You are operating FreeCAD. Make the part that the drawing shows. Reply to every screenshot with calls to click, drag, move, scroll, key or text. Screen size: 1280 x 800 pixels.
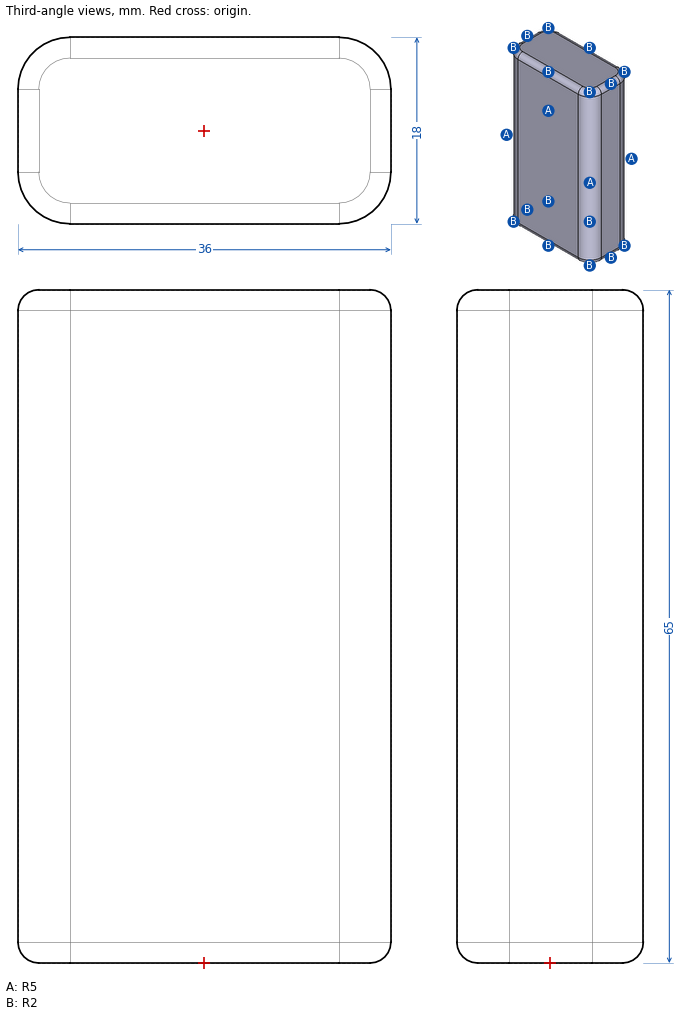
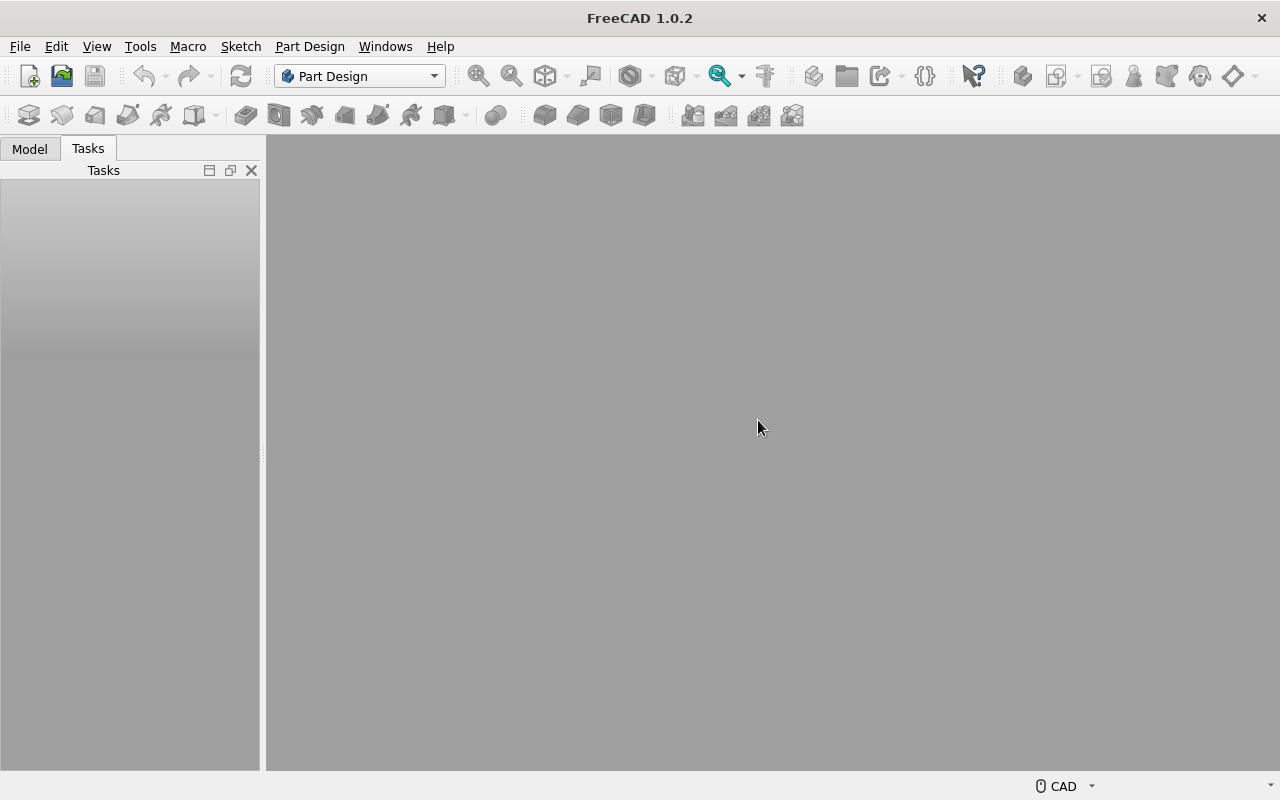
click(29, 76)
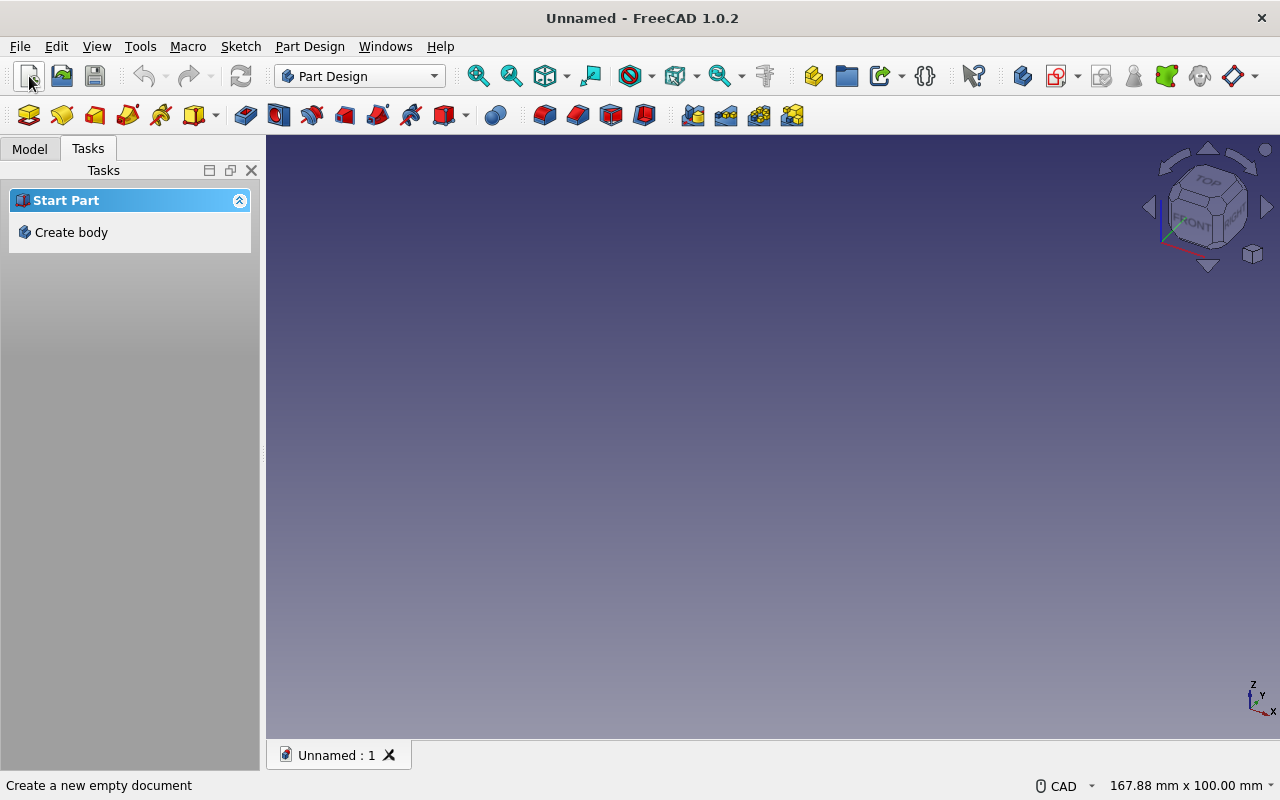
click(1056, 76)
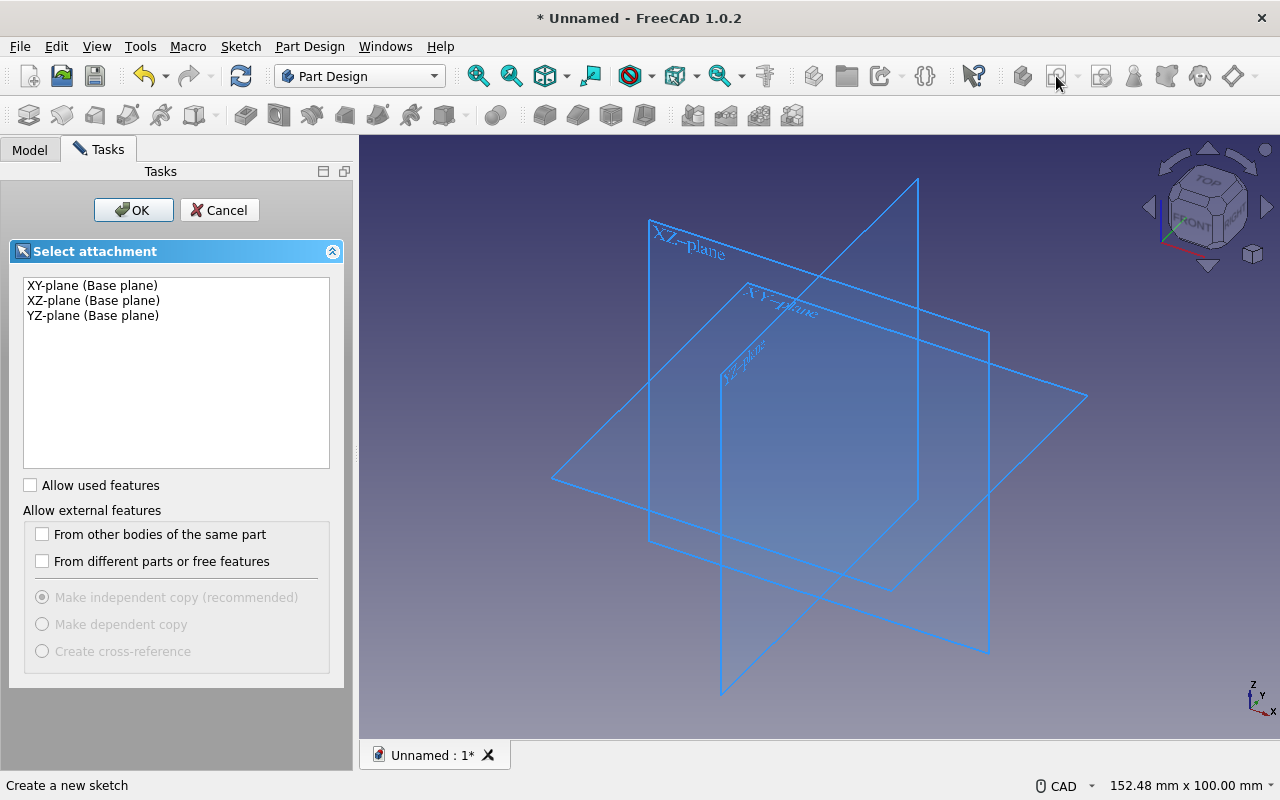
click(84, 286)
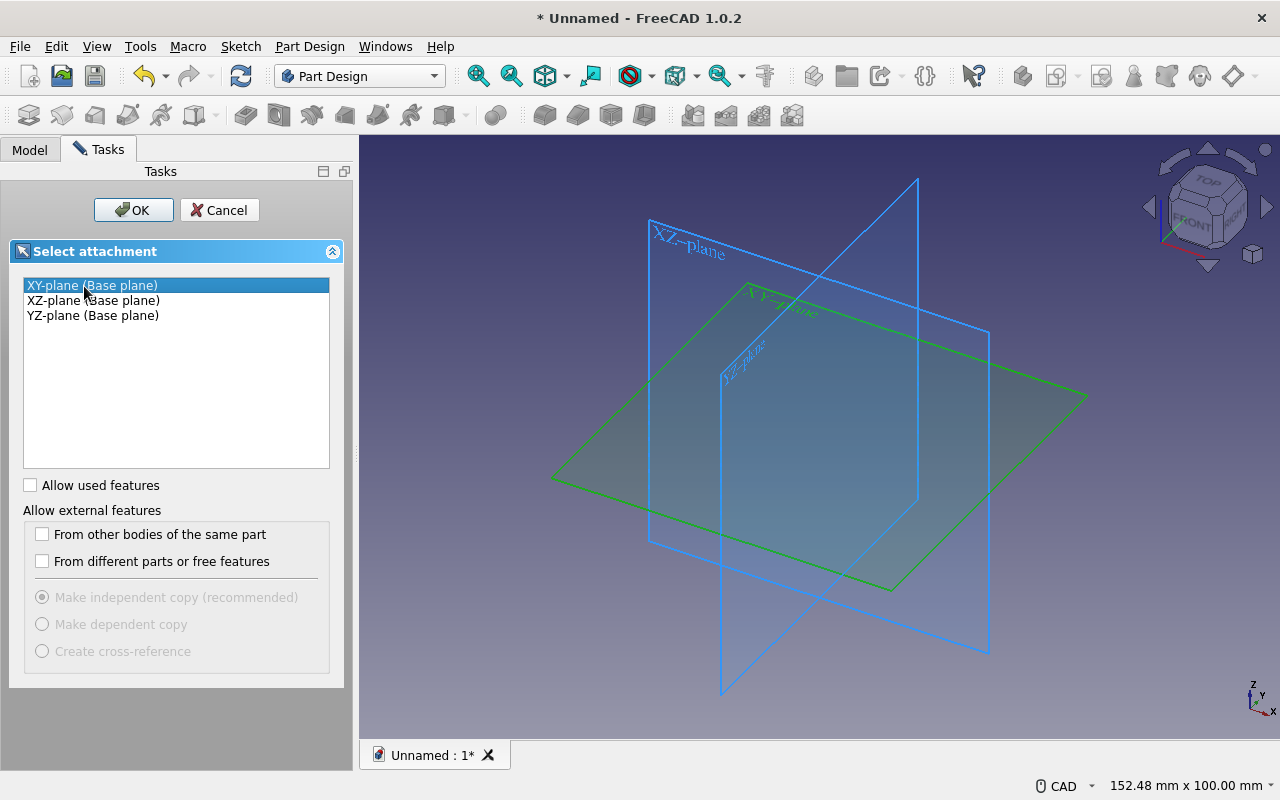
click(134, 210)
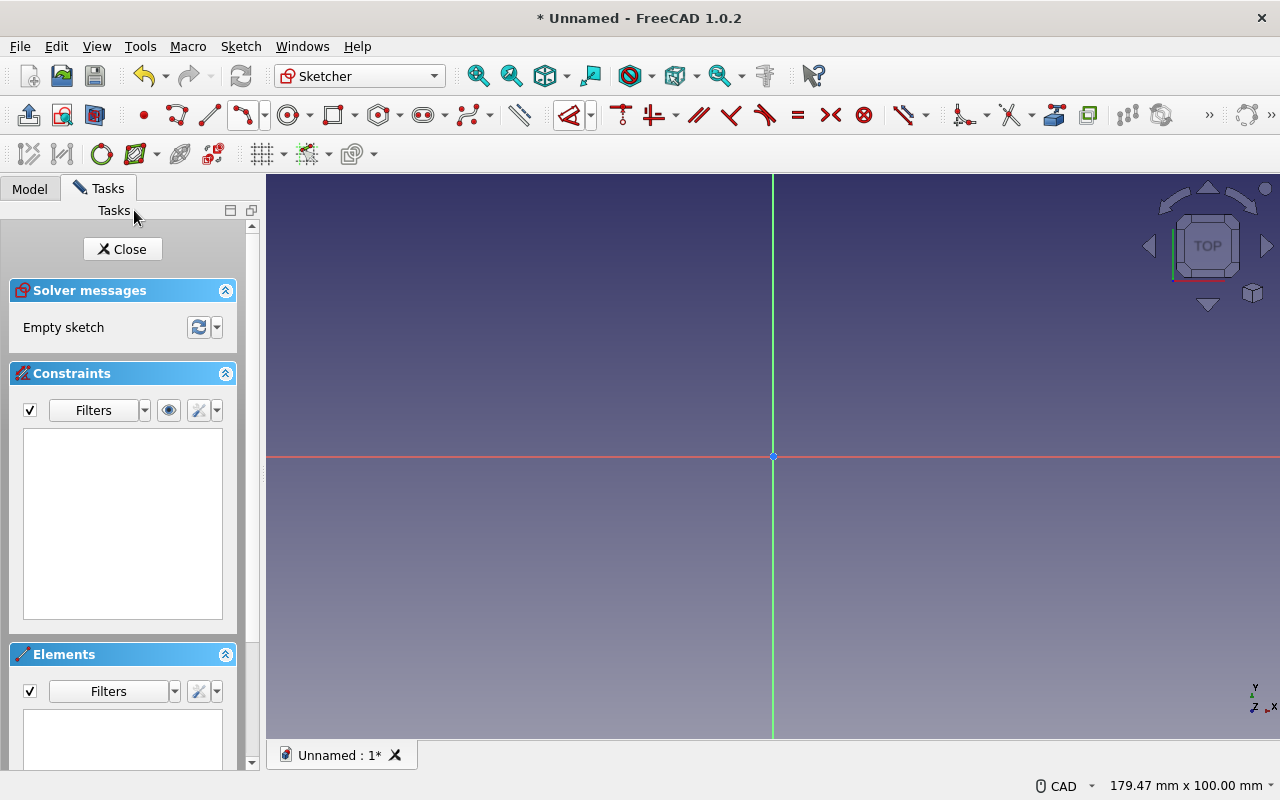
scroll(813, 456, up, 5)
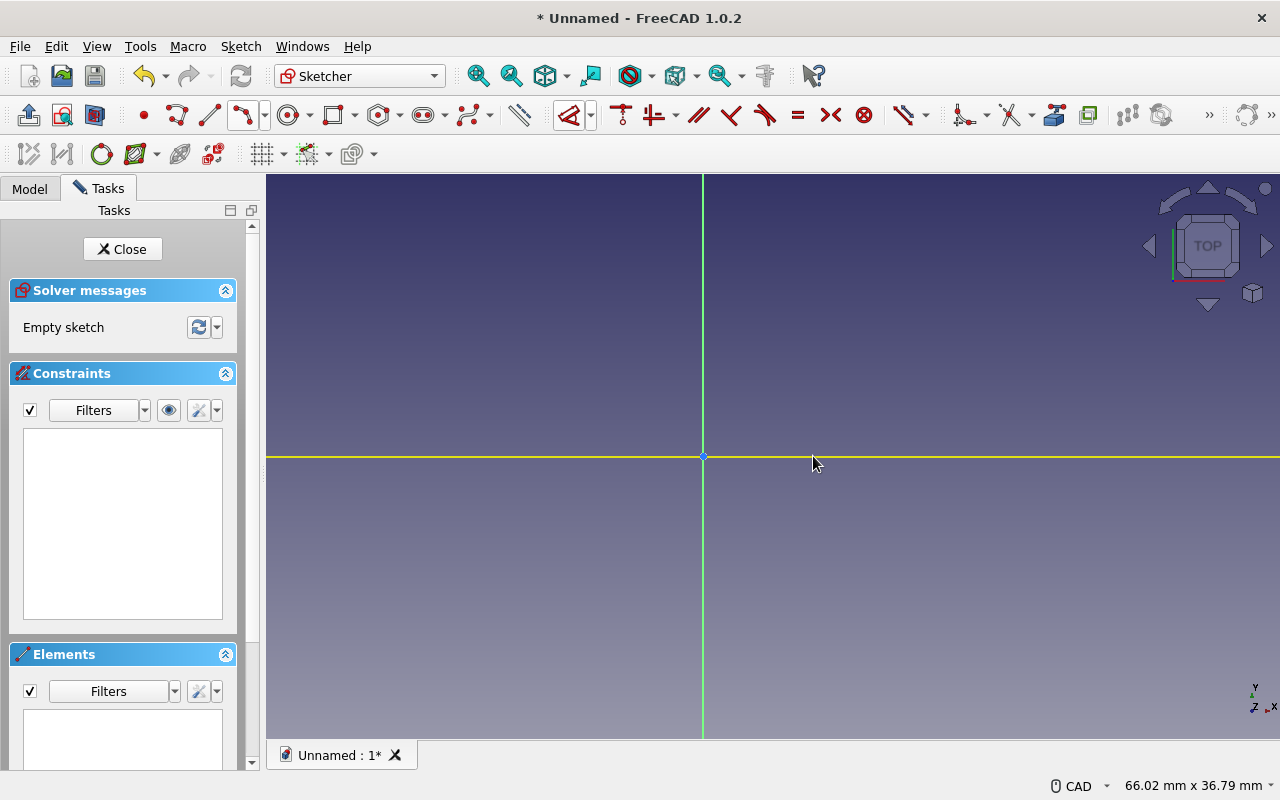
key(g)
key(v)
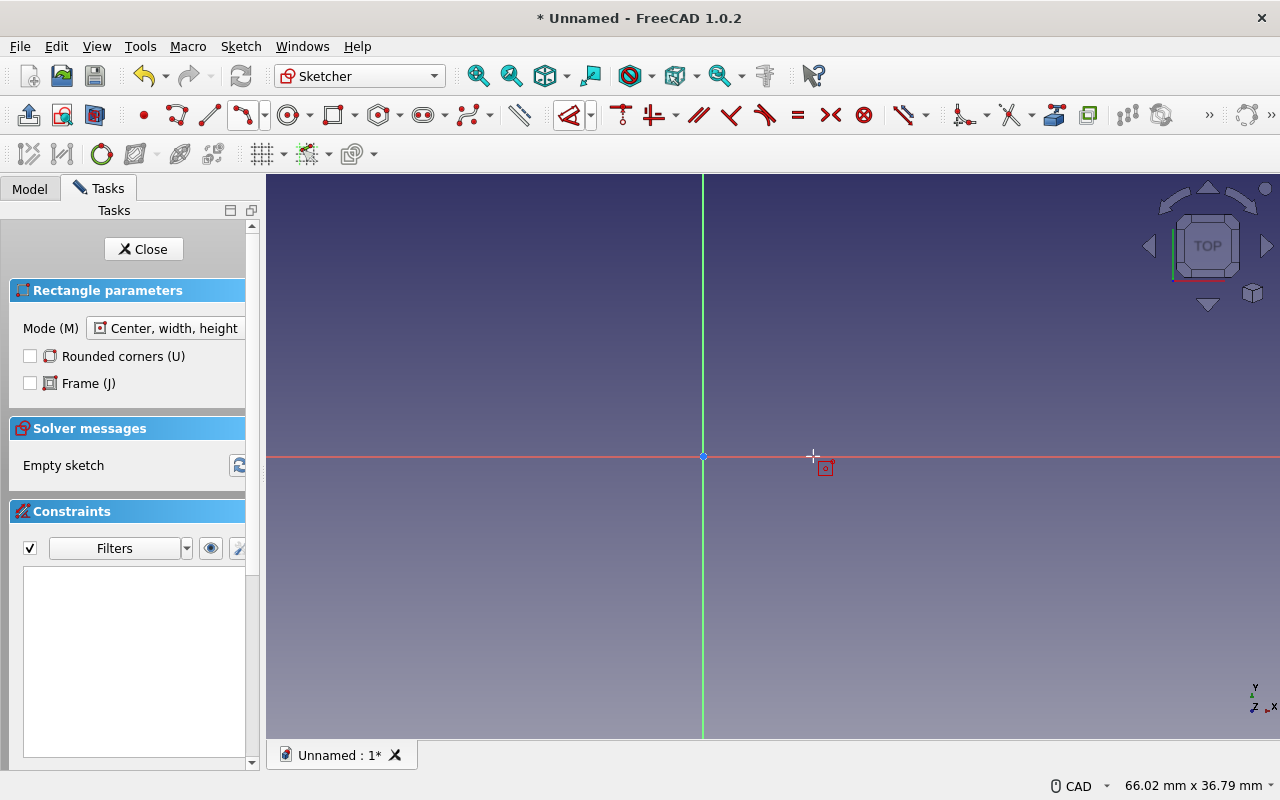
click(703, 456)
click(980, 318)
key(Escape)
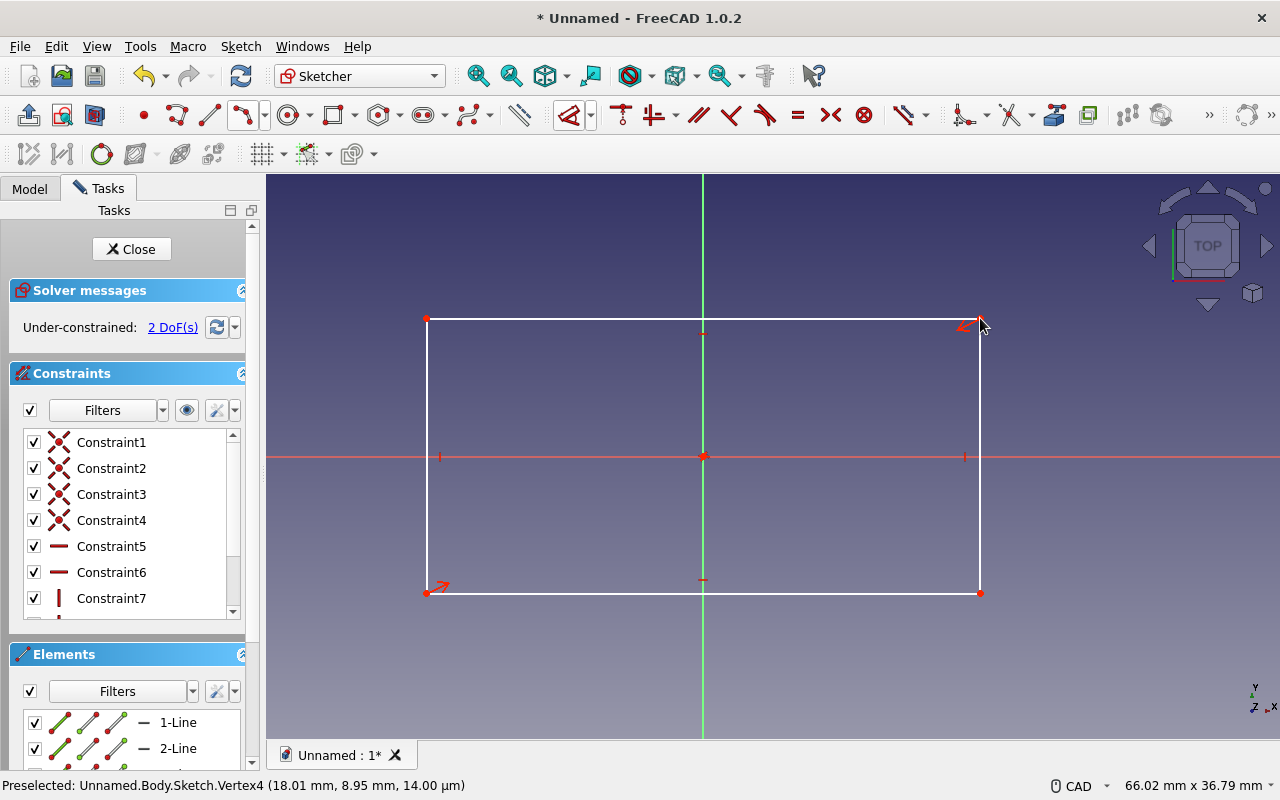
click(593, 594)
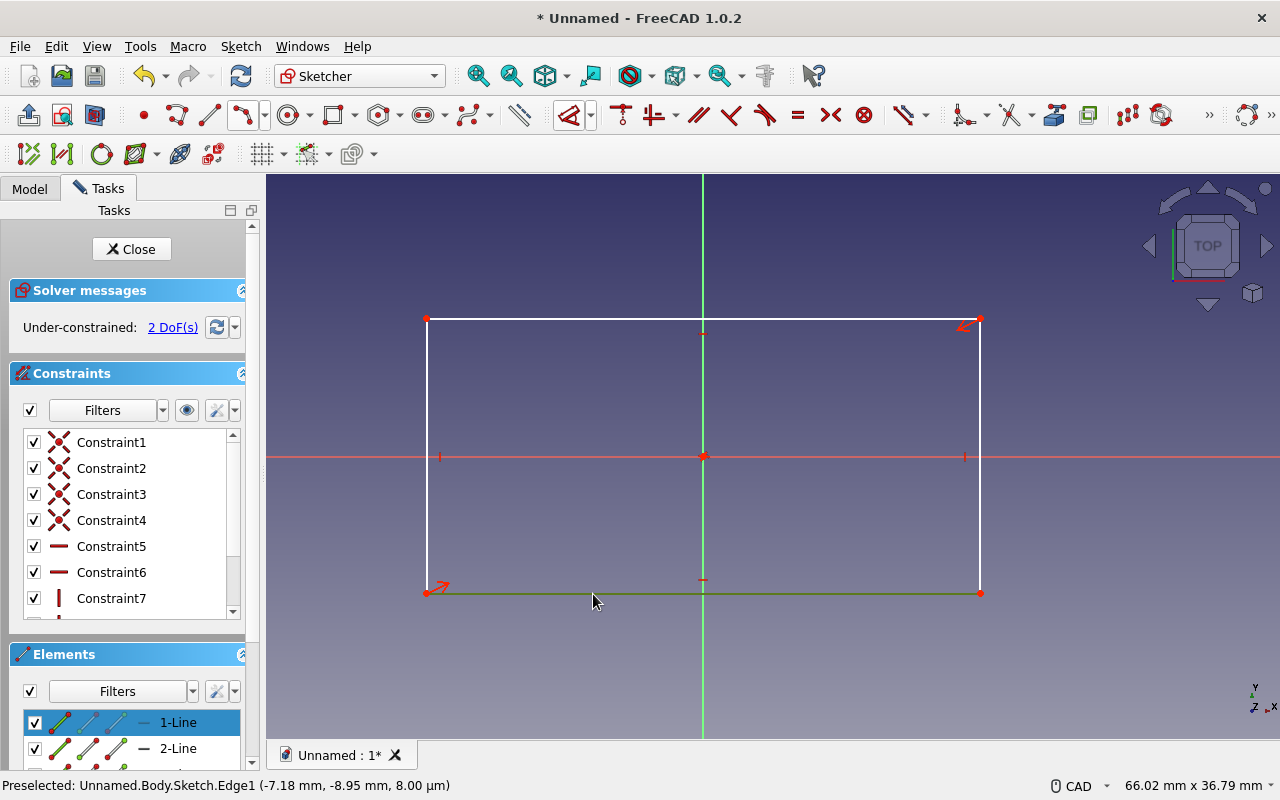
click(590, 116)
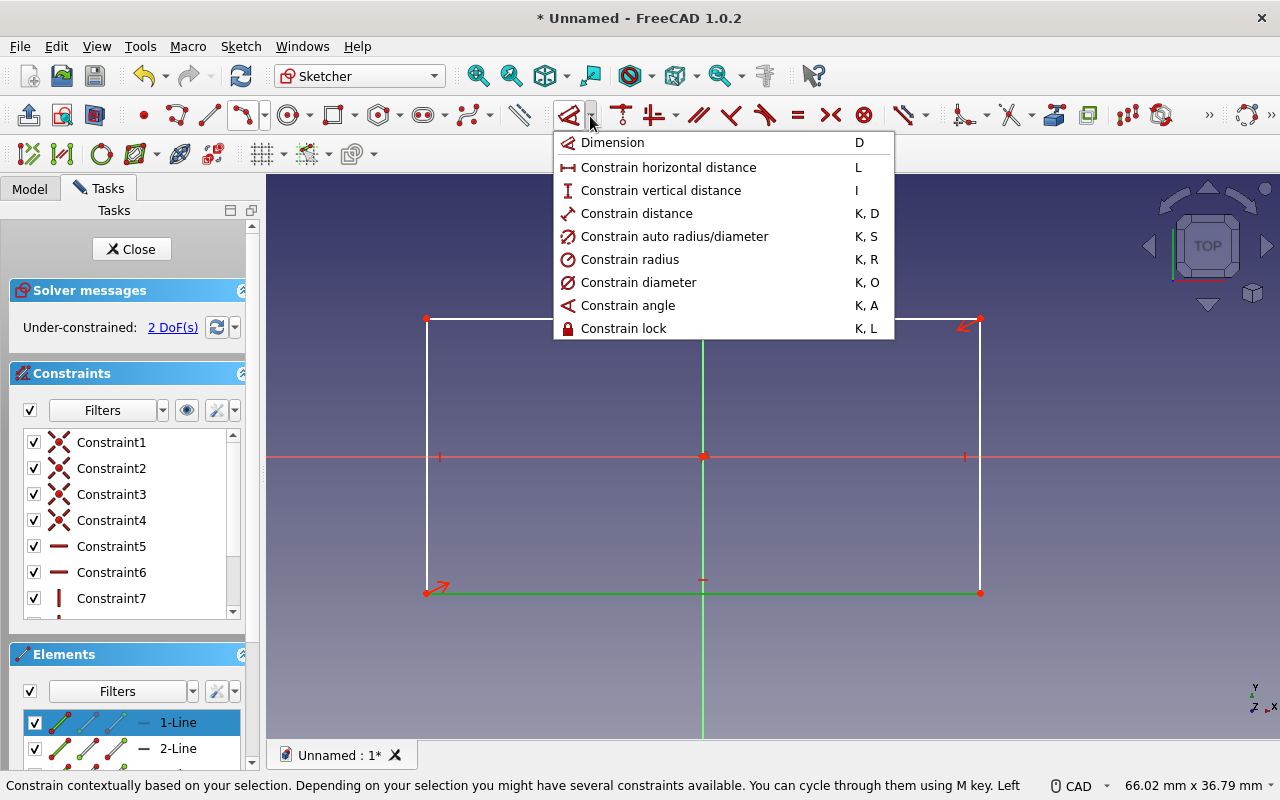
click(724, 168)